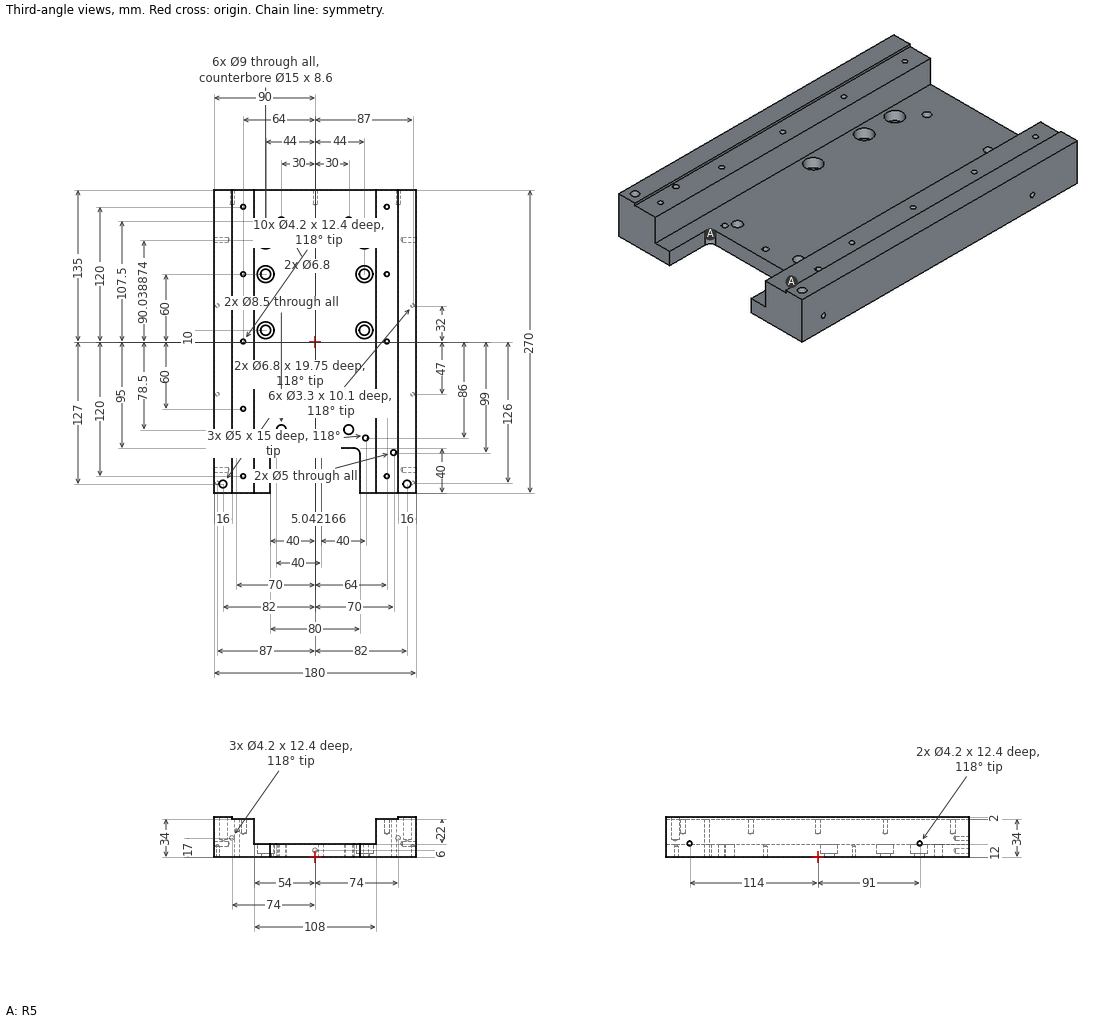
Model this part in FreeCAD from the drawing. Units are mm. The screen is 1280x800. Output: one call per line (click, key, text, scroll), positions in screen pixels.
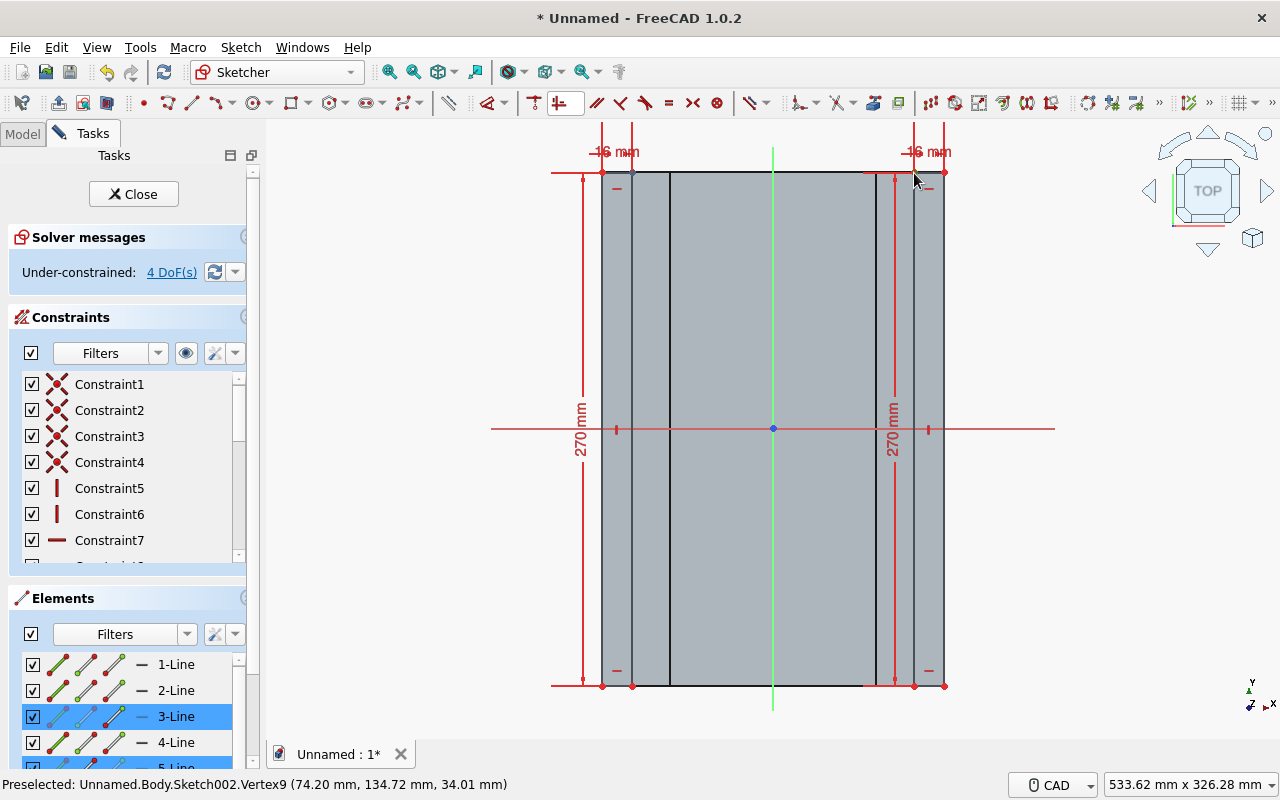
click(773, 671)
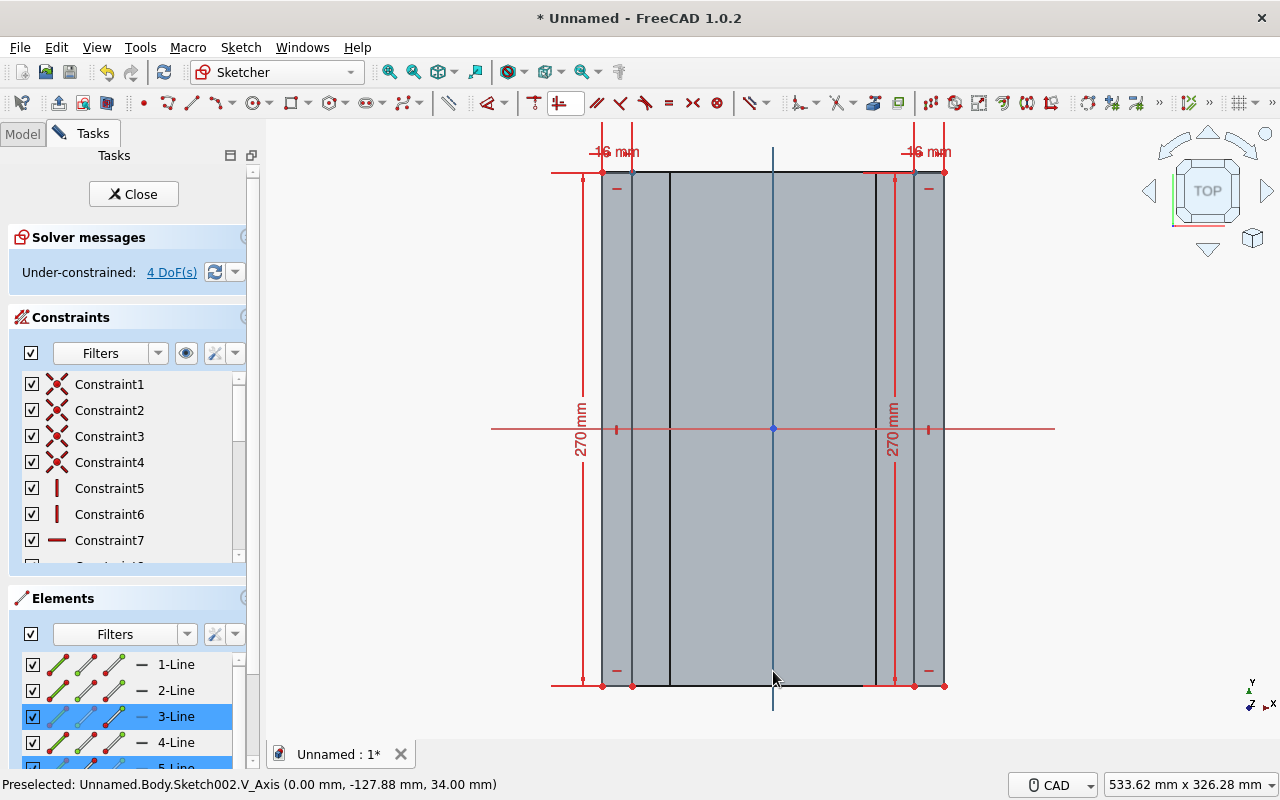
click(694, 104)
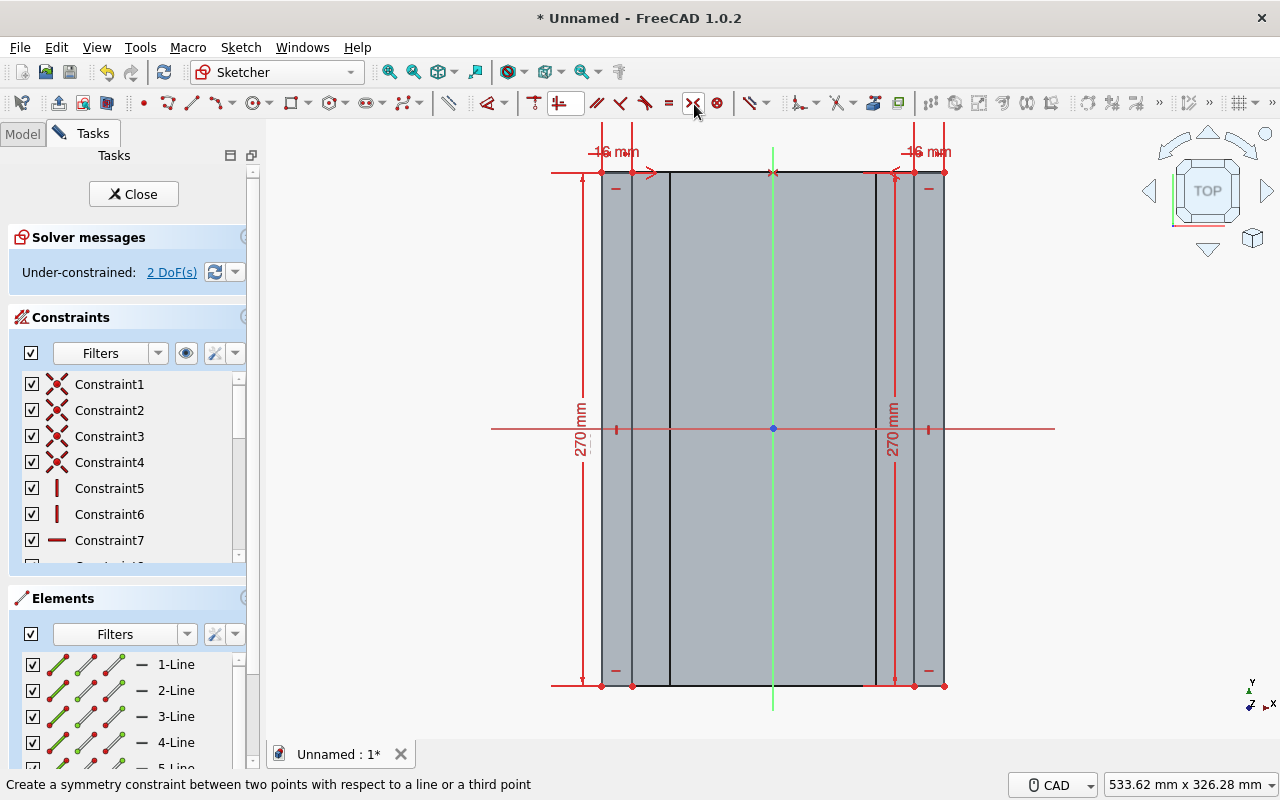
click(488, 104)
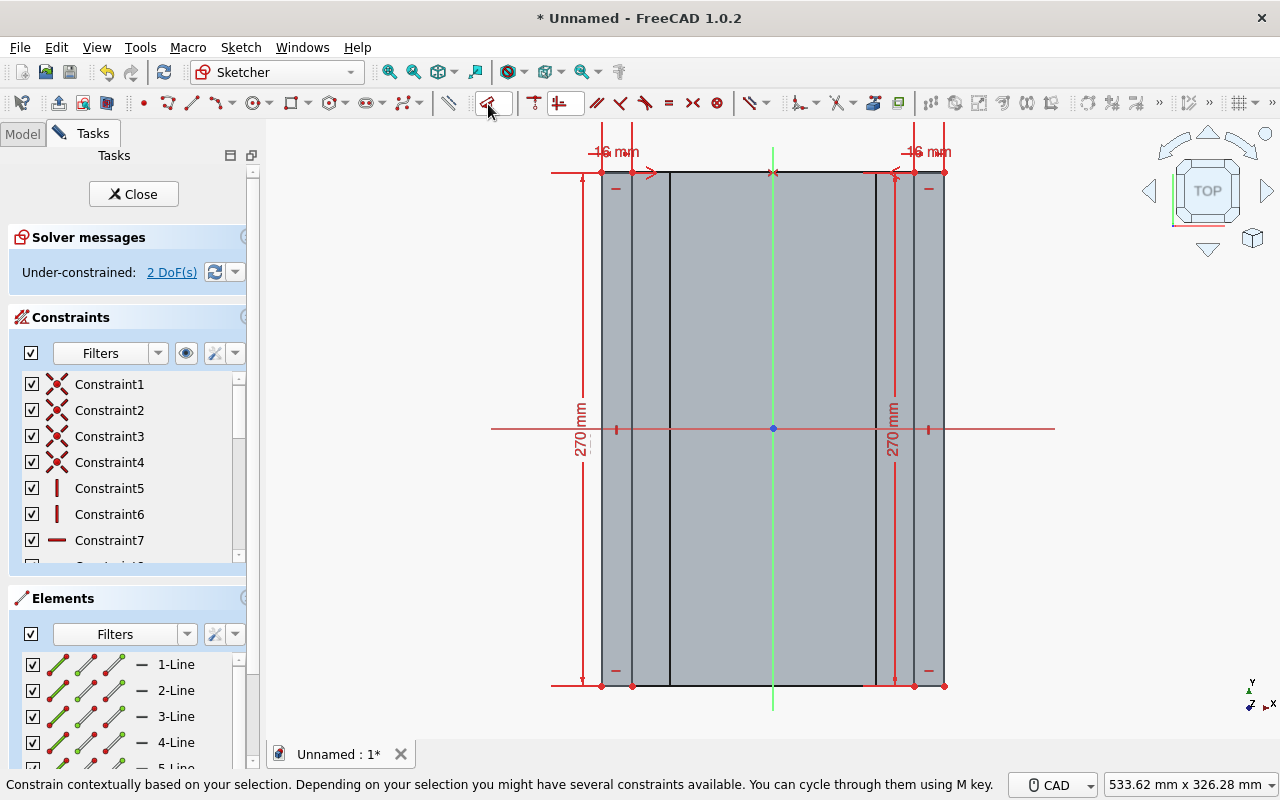
click(602, 173)
click(687, 463)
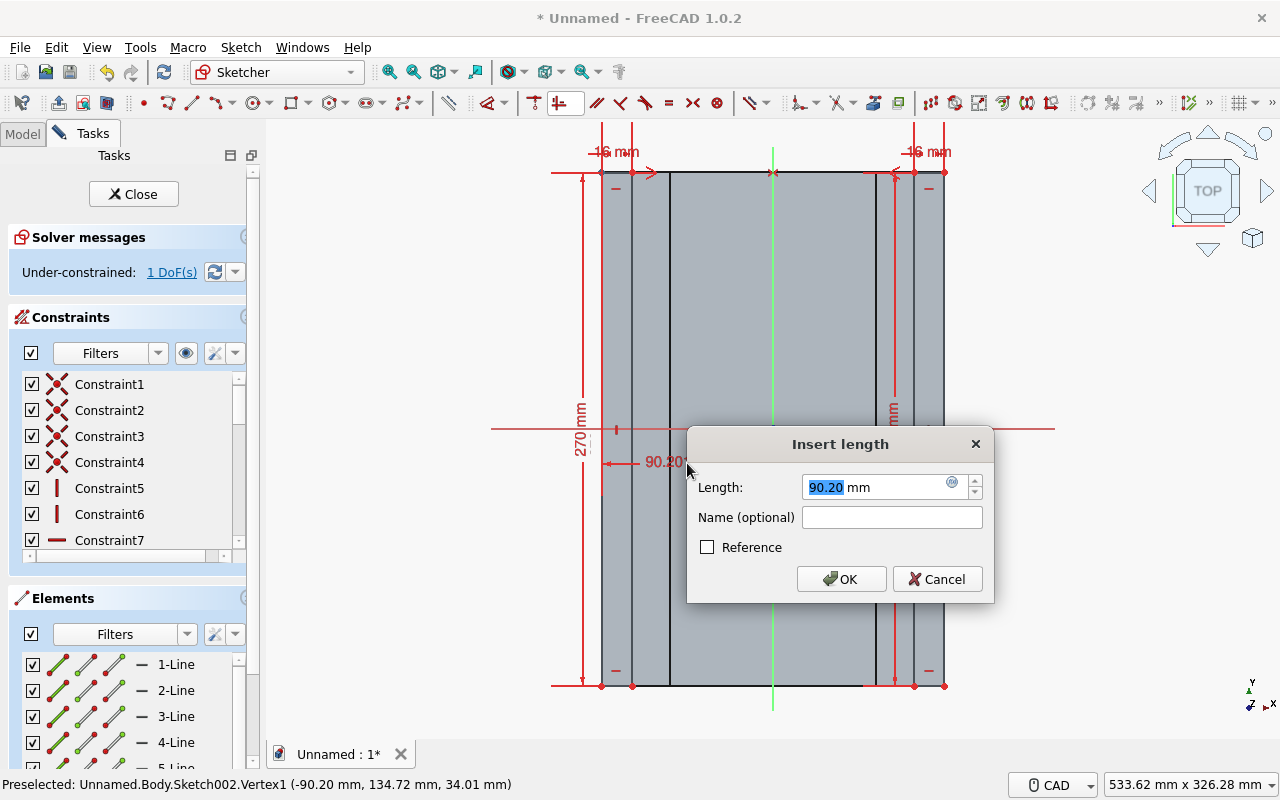
text(90)
key(Return)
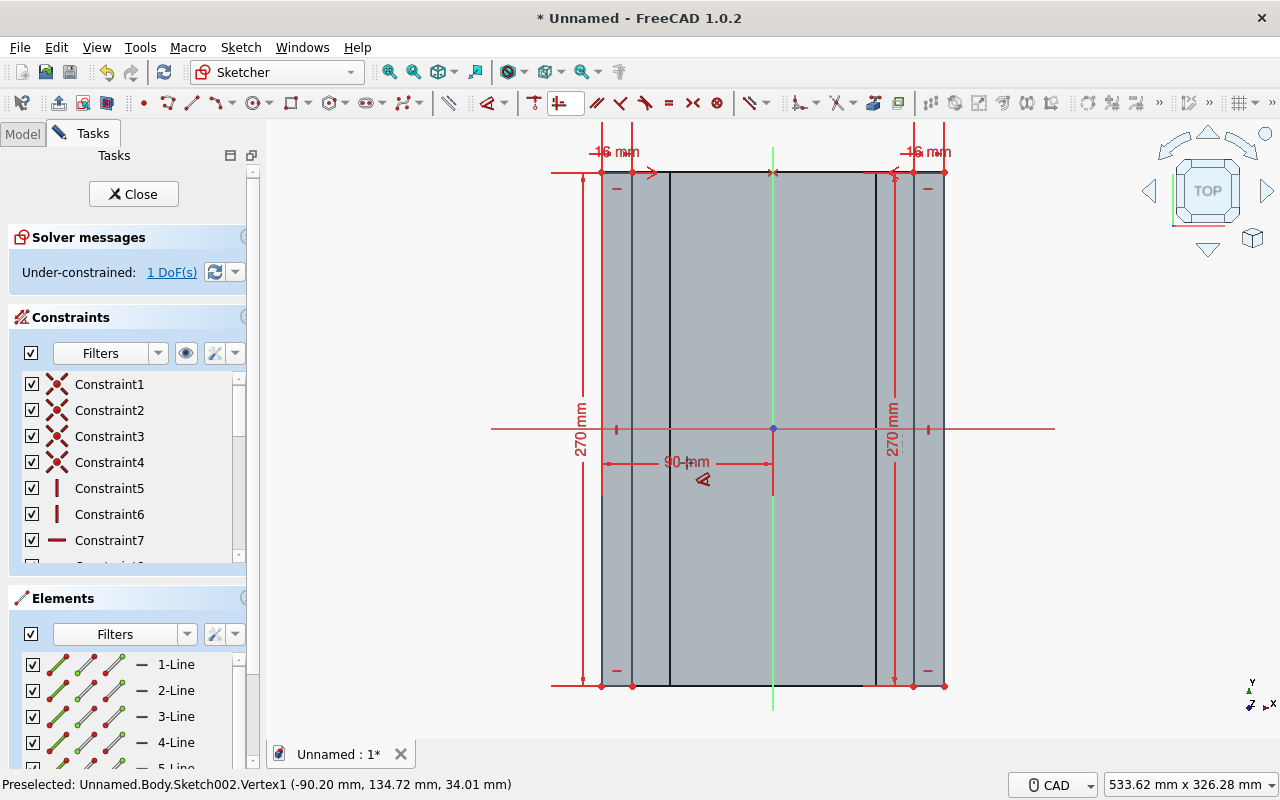
click(602, 173)
click(568, 301)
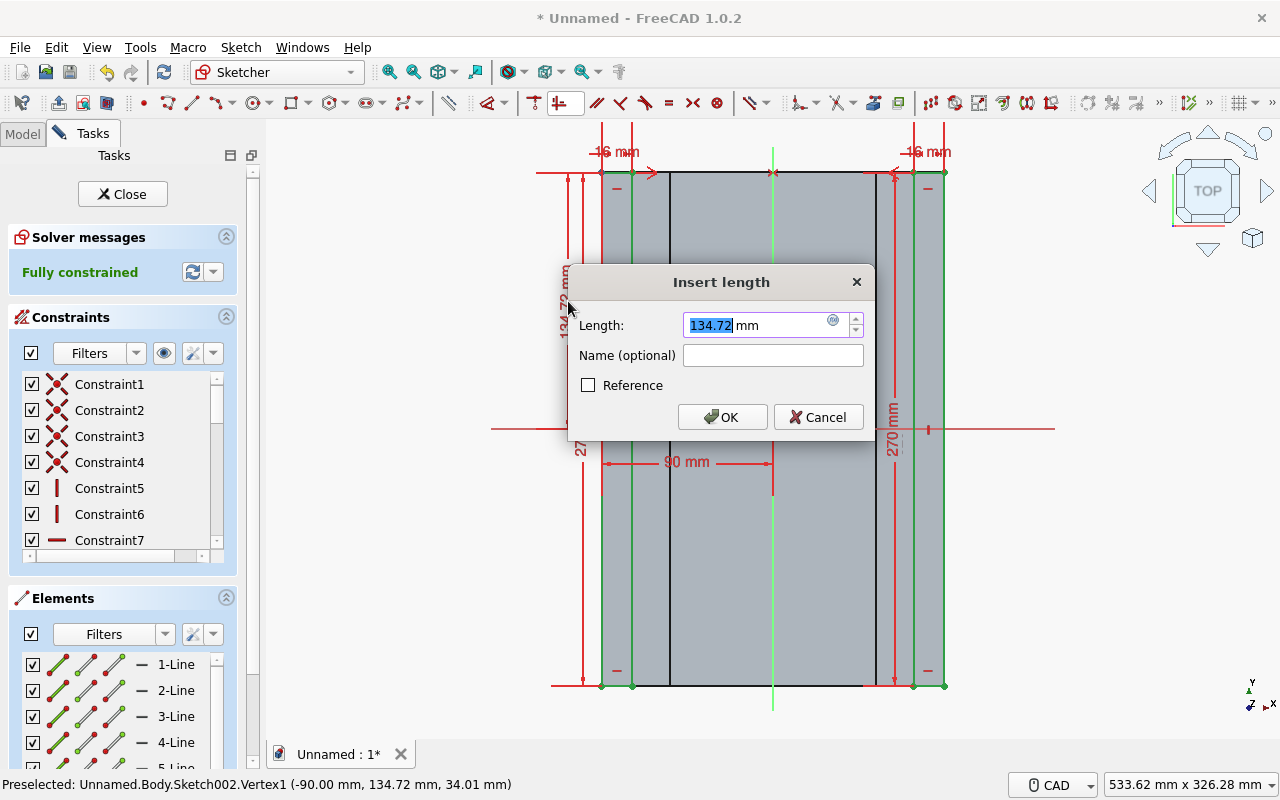
text(135)
key(Return)
key(Escape)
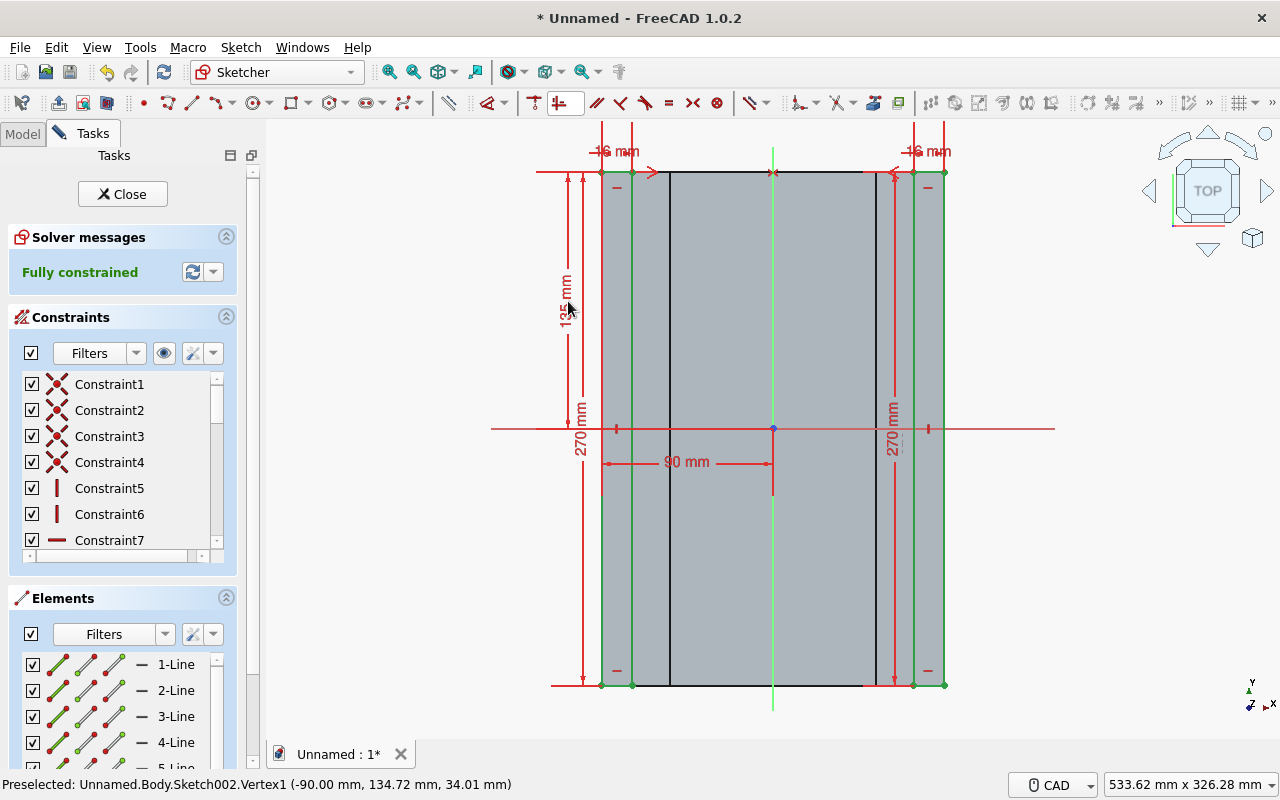
click(123, 194)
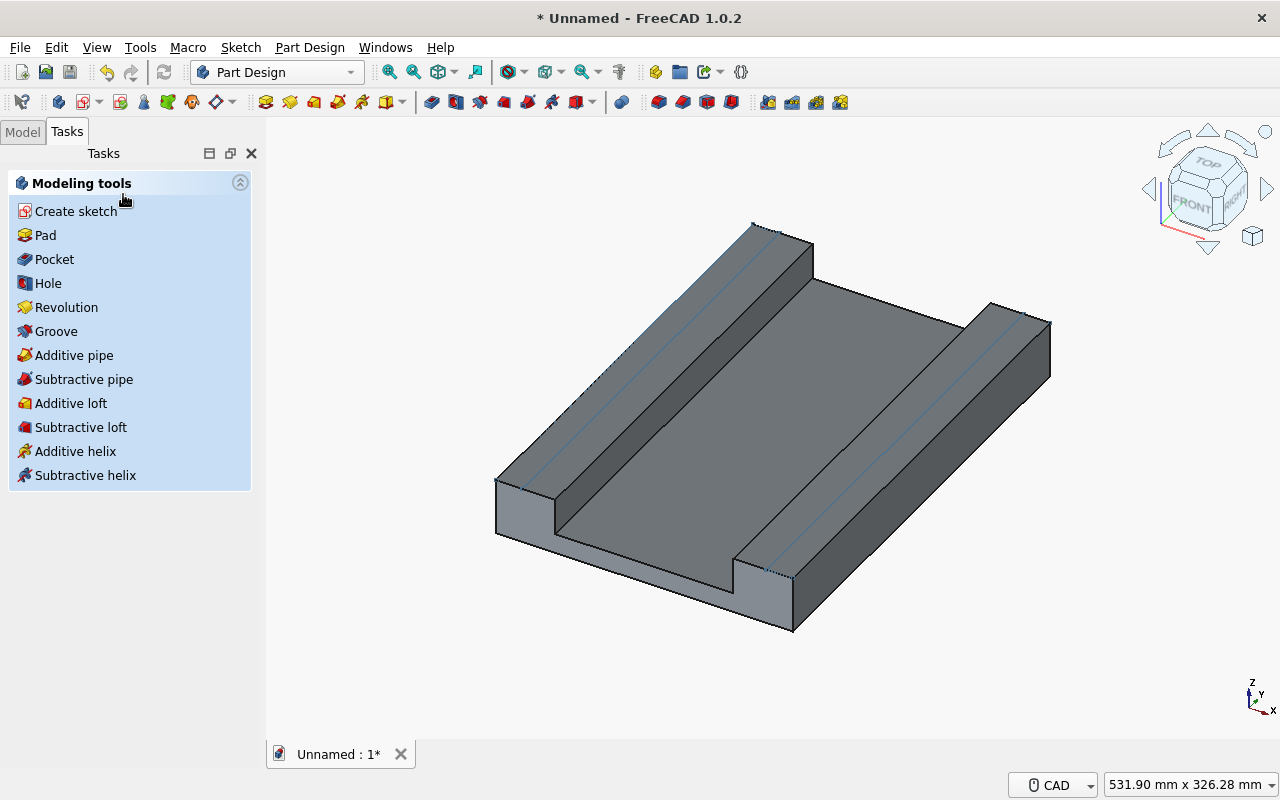
click(266, 102)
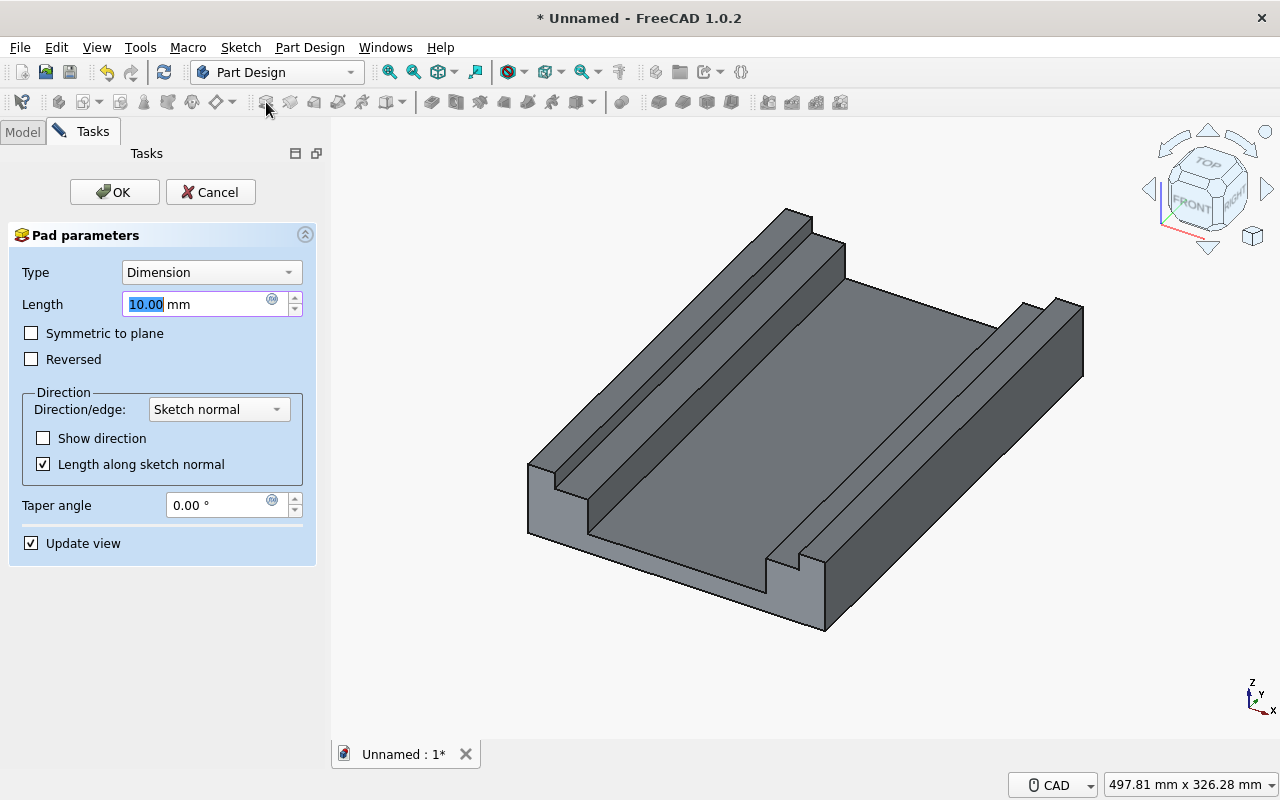
text(2)
key(Tab)